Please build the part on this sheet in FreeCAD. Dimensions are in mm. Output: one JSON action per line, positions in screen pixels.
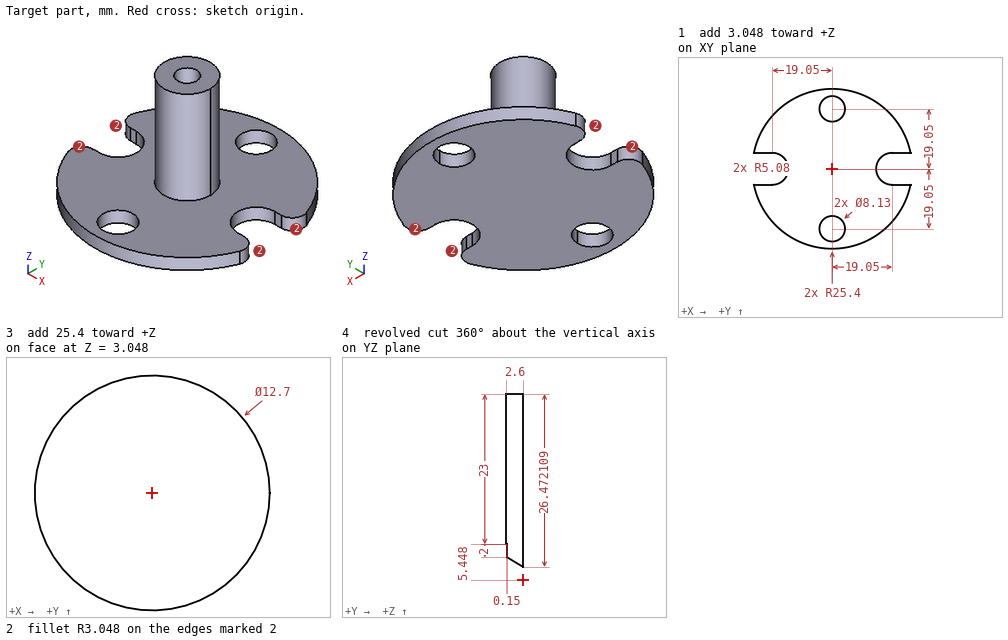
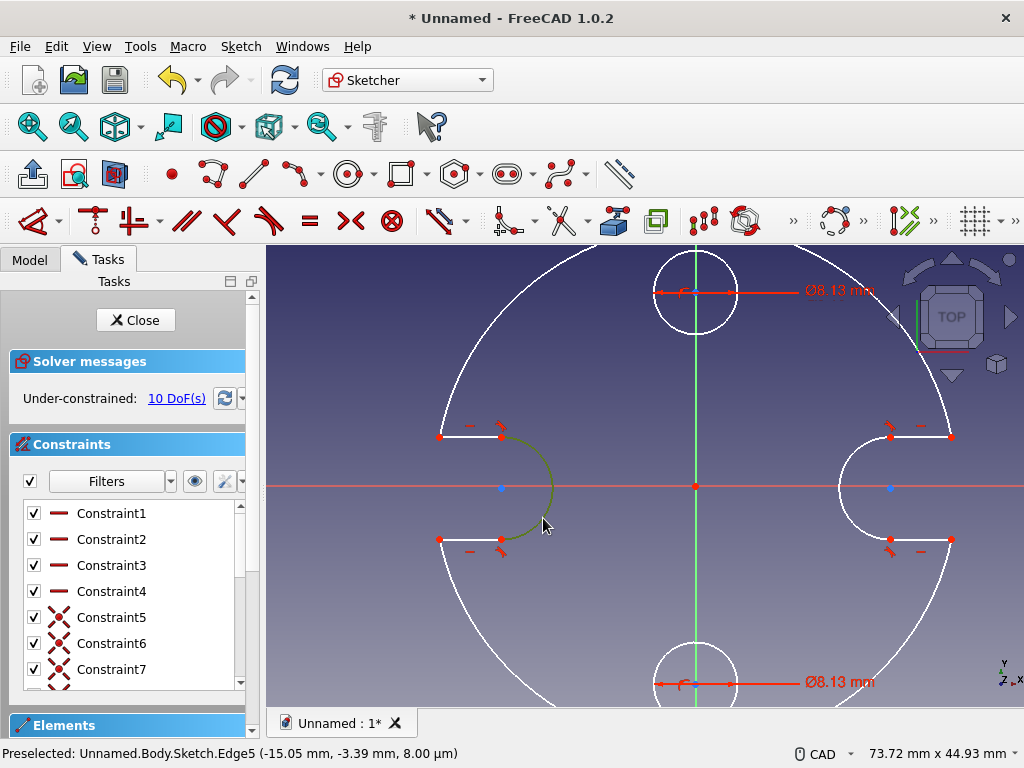
{"action": "left_click", "coordinate": [849, 458]}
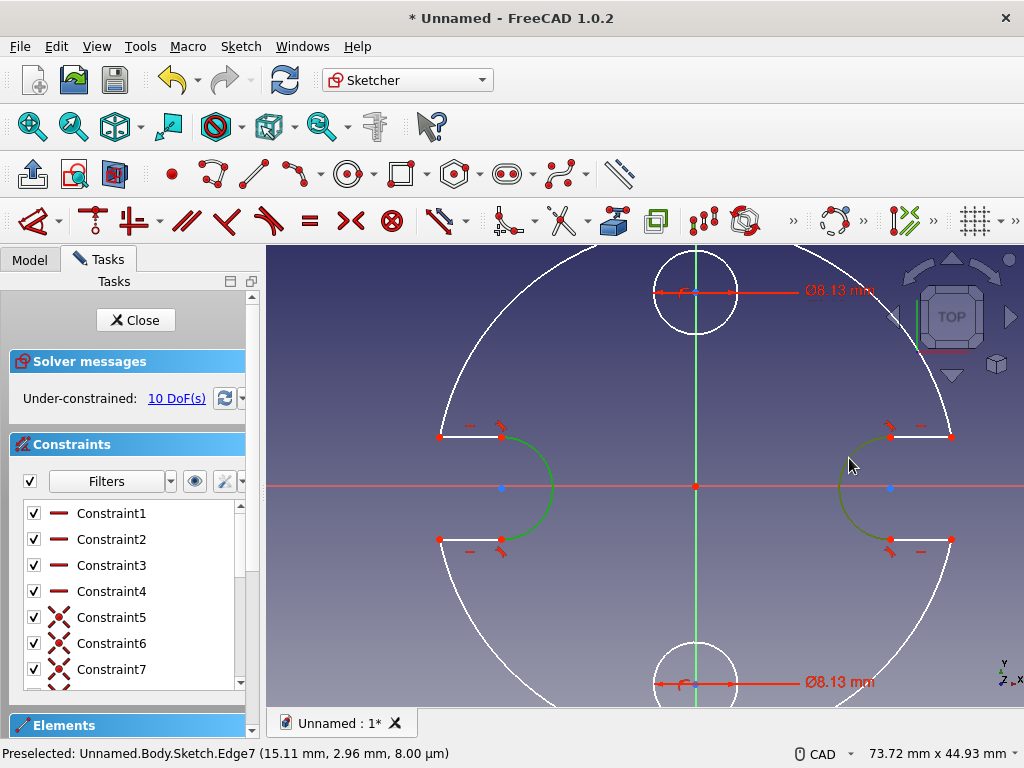
{"action": "left_click", "coordinate": [310, 222]}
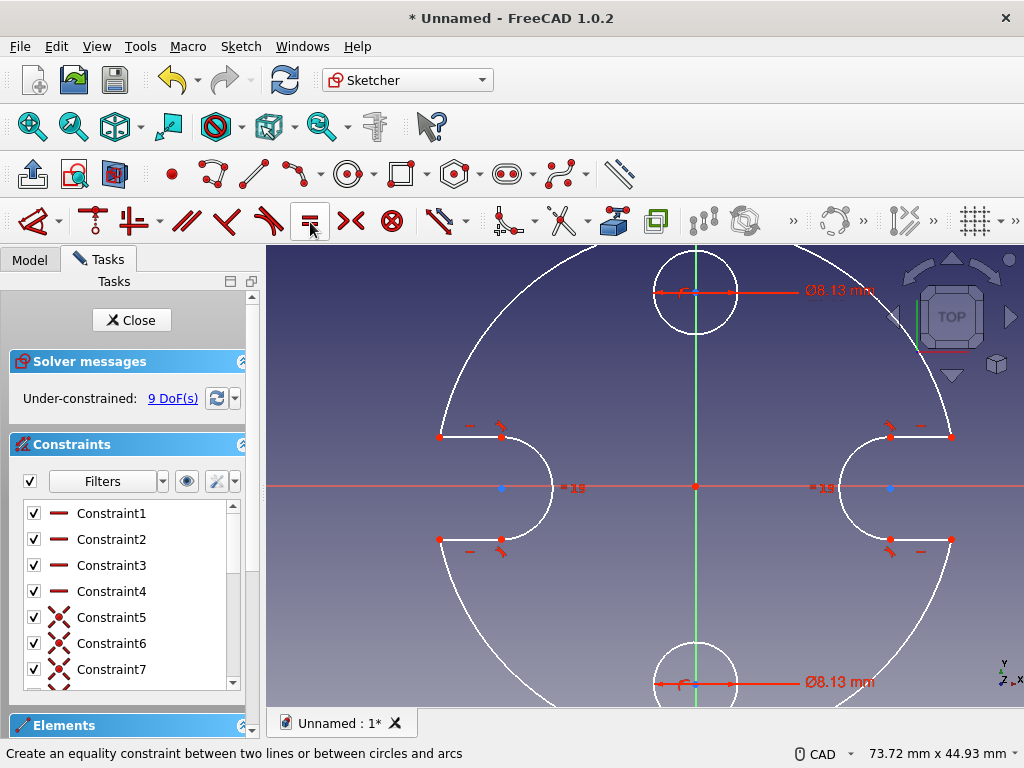
{"action": "left_click", "coordinate": [505, 665]}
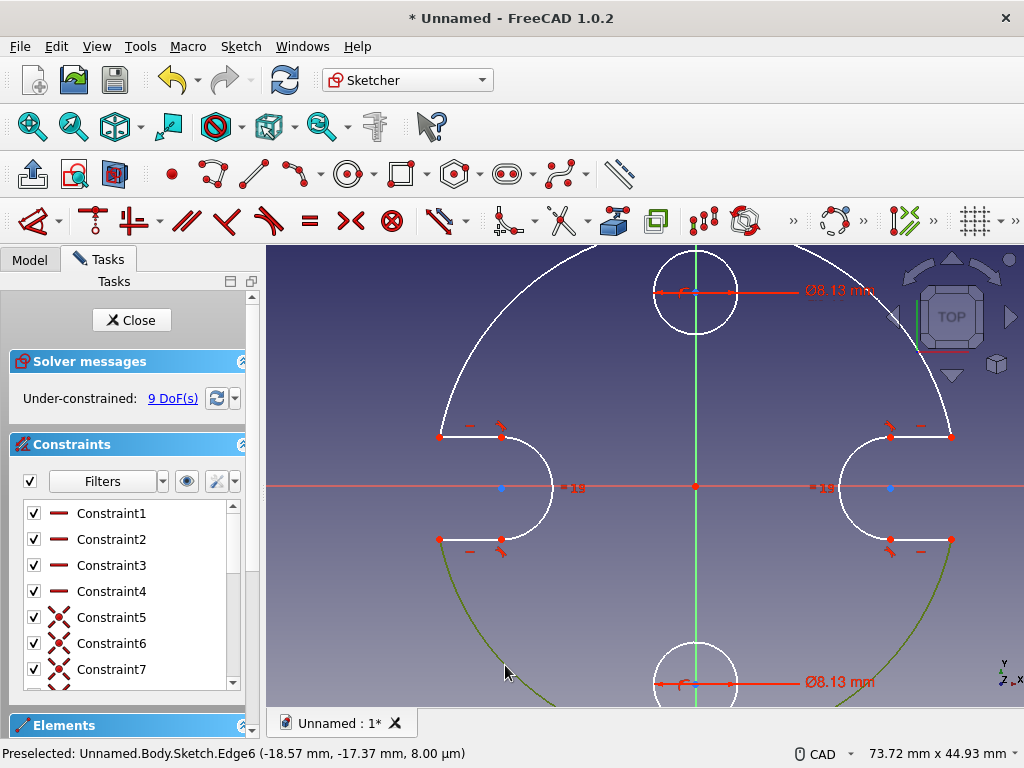
{"action": "left_click", "coordinate": [504, 310]}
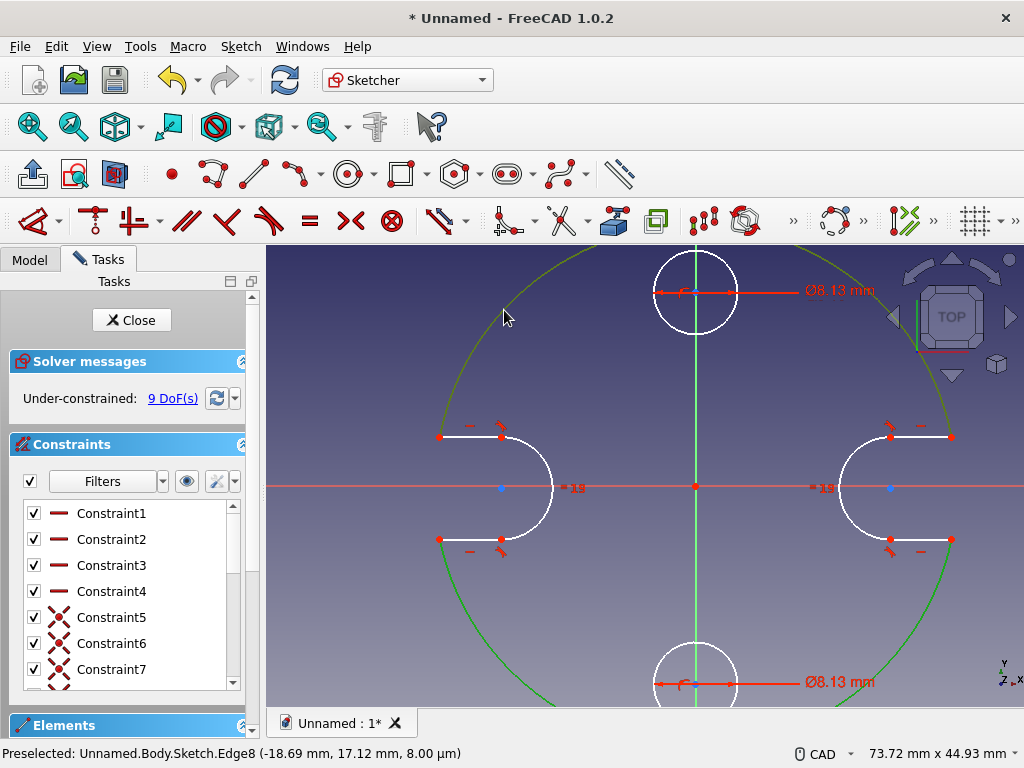
{"action": "left_click", "coordinate": [310, 222]}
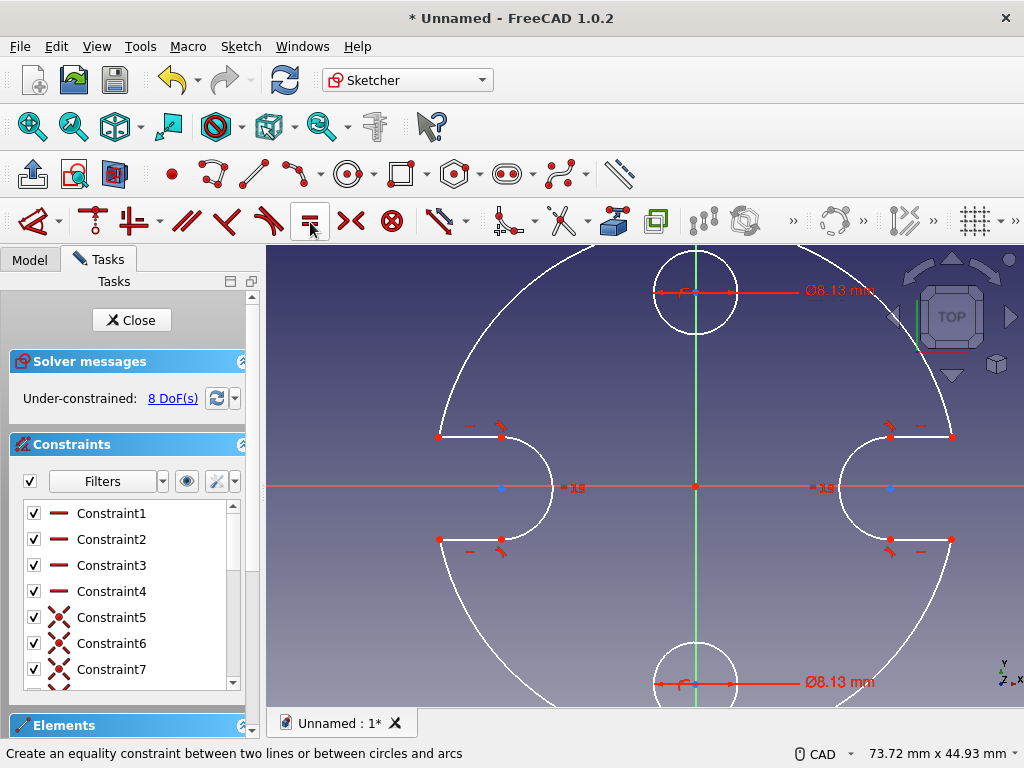
{"action": "left_click", "coordinate": [501, 488]}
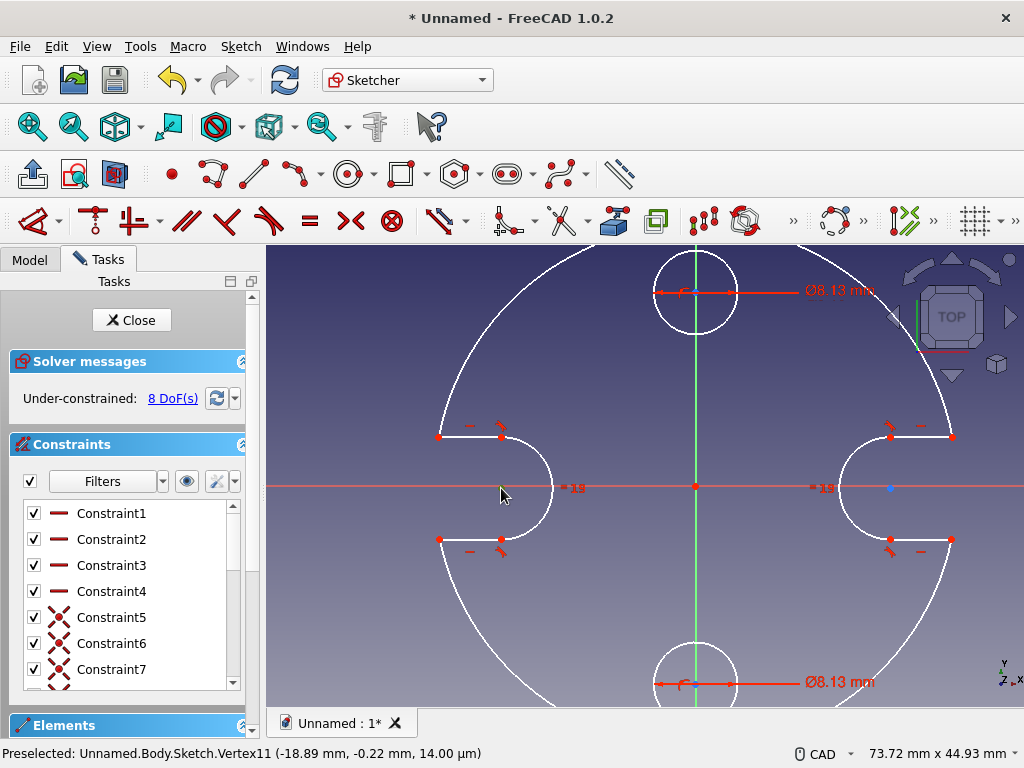
{"action": "left_click", "coordinate": [334, 486]}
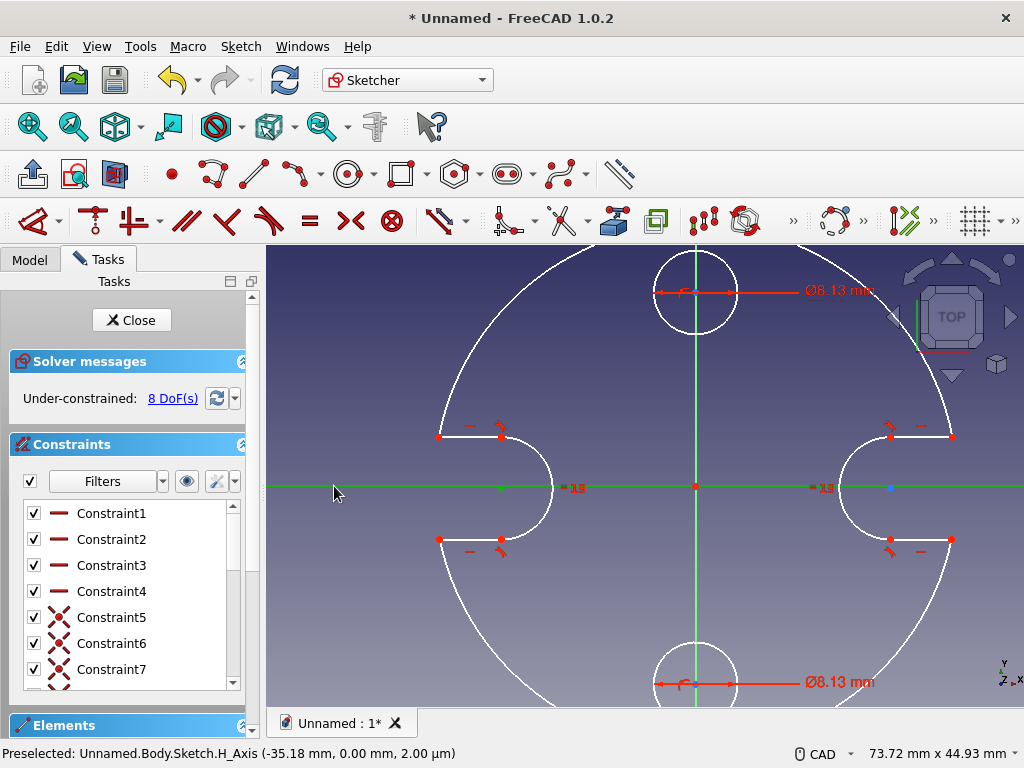
{"action": "left_click", "coordinate": [93, 222]}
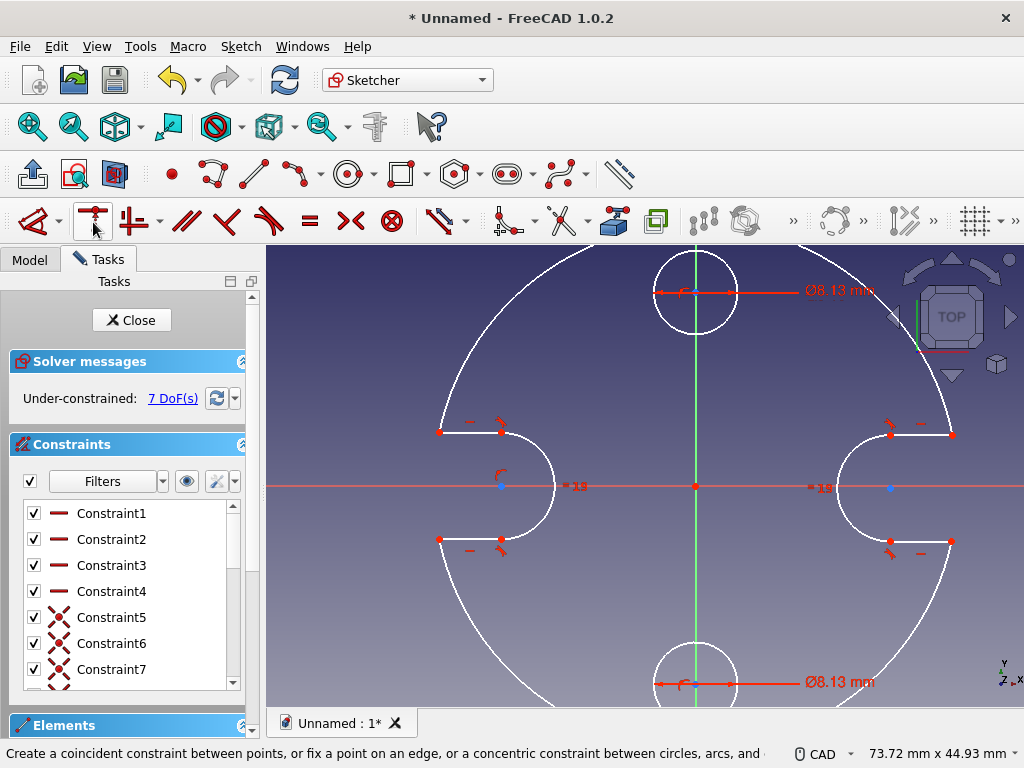
{"action": "scroll", "coordinate": [432, 464], "scroll_direction": "down", "scroll_amount": 3}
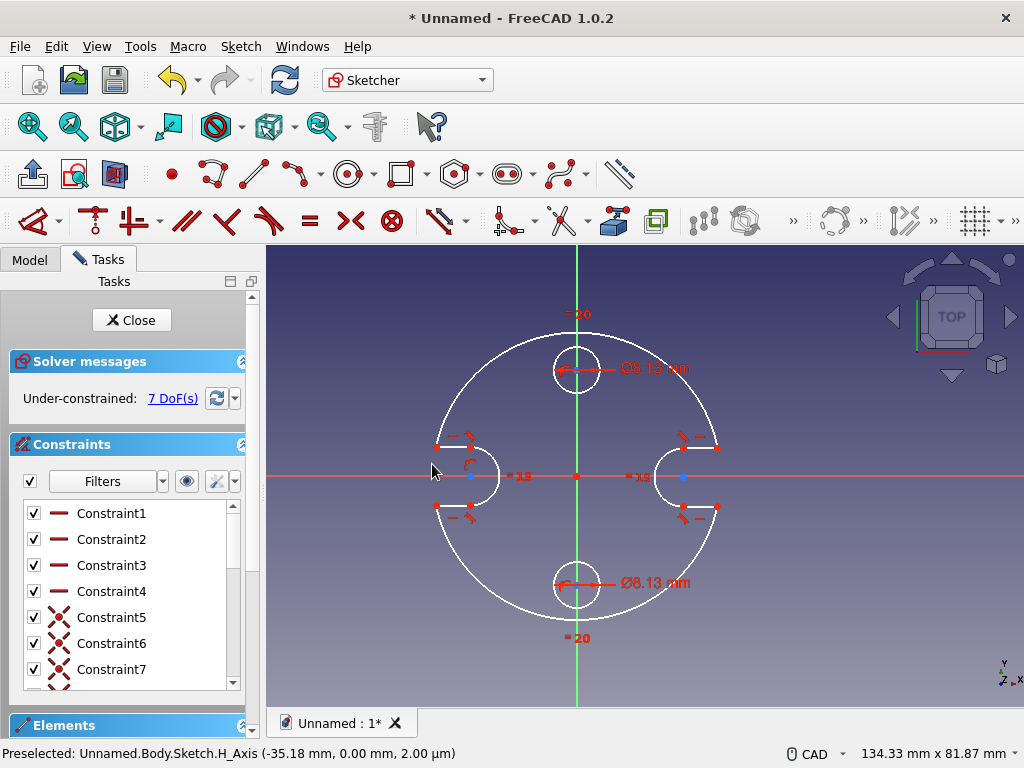
{"action": "left_click", "coordinate": [684, 478]}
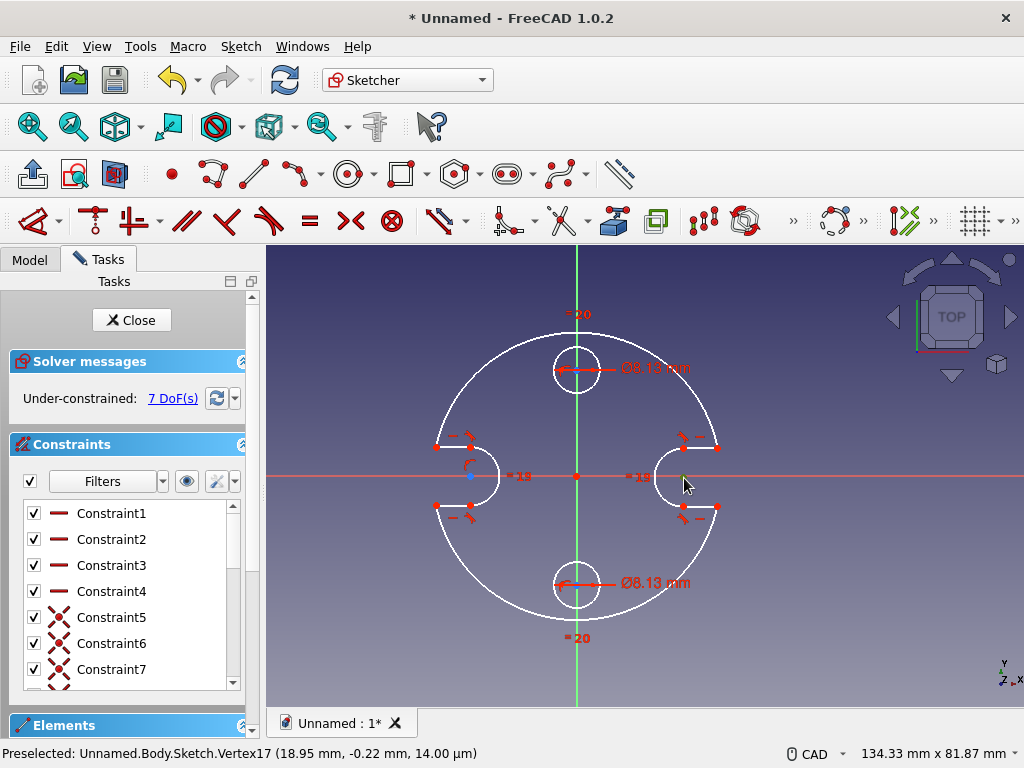
{"action": "left_click", "coordinate": [334, 476]}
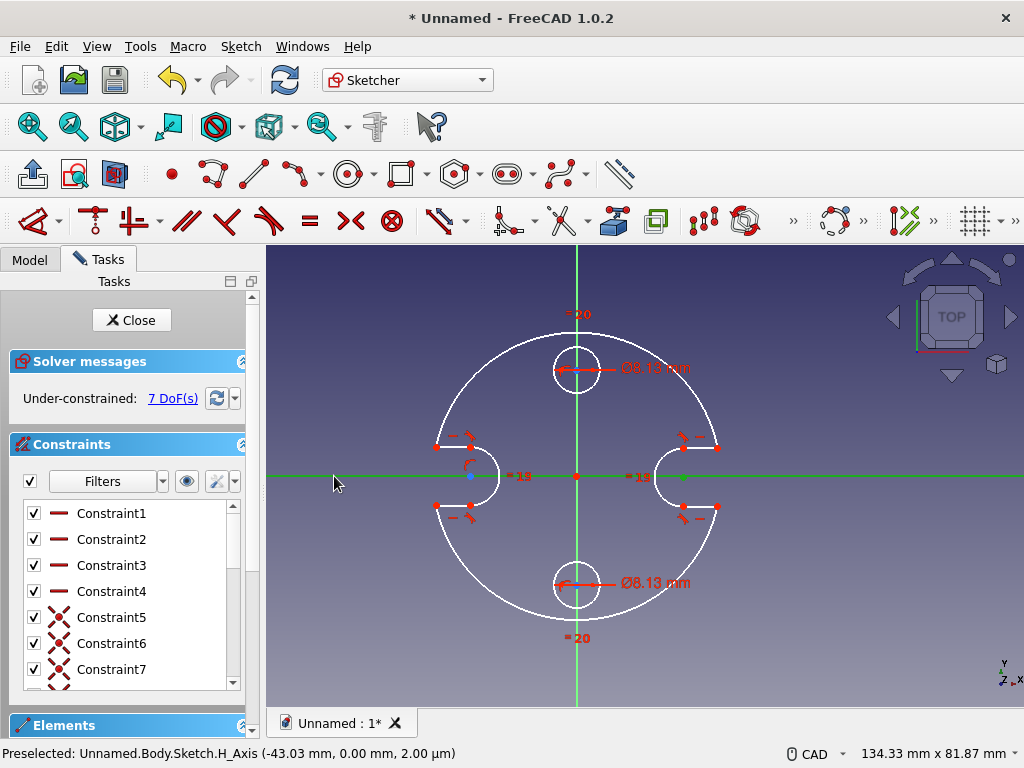
{"action": "left_click", "coordinate": [93, 222]}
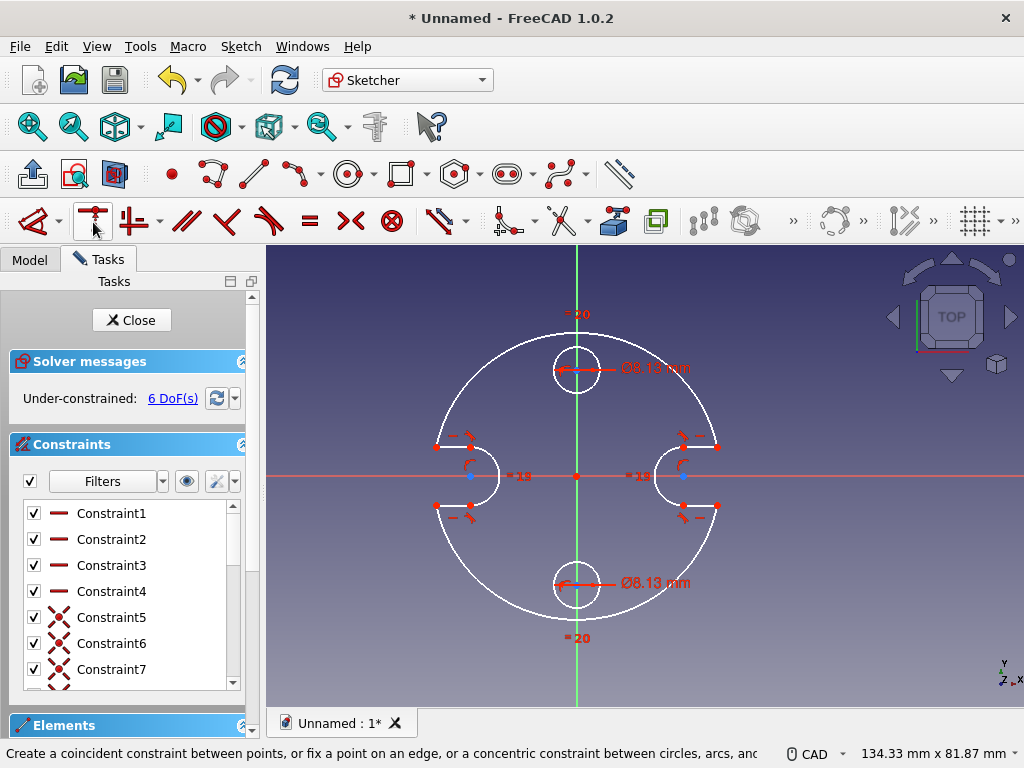
{"action": "left_click", "coordinate": [32, 222]}